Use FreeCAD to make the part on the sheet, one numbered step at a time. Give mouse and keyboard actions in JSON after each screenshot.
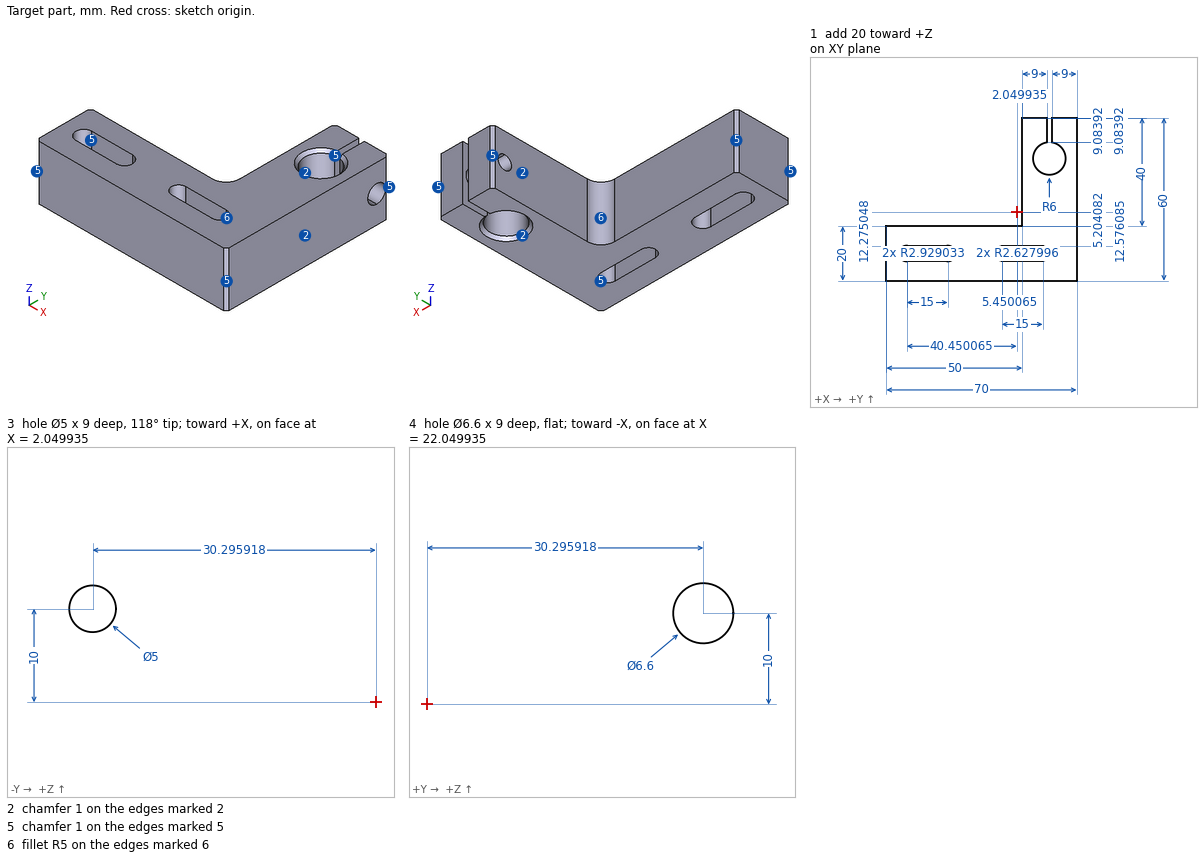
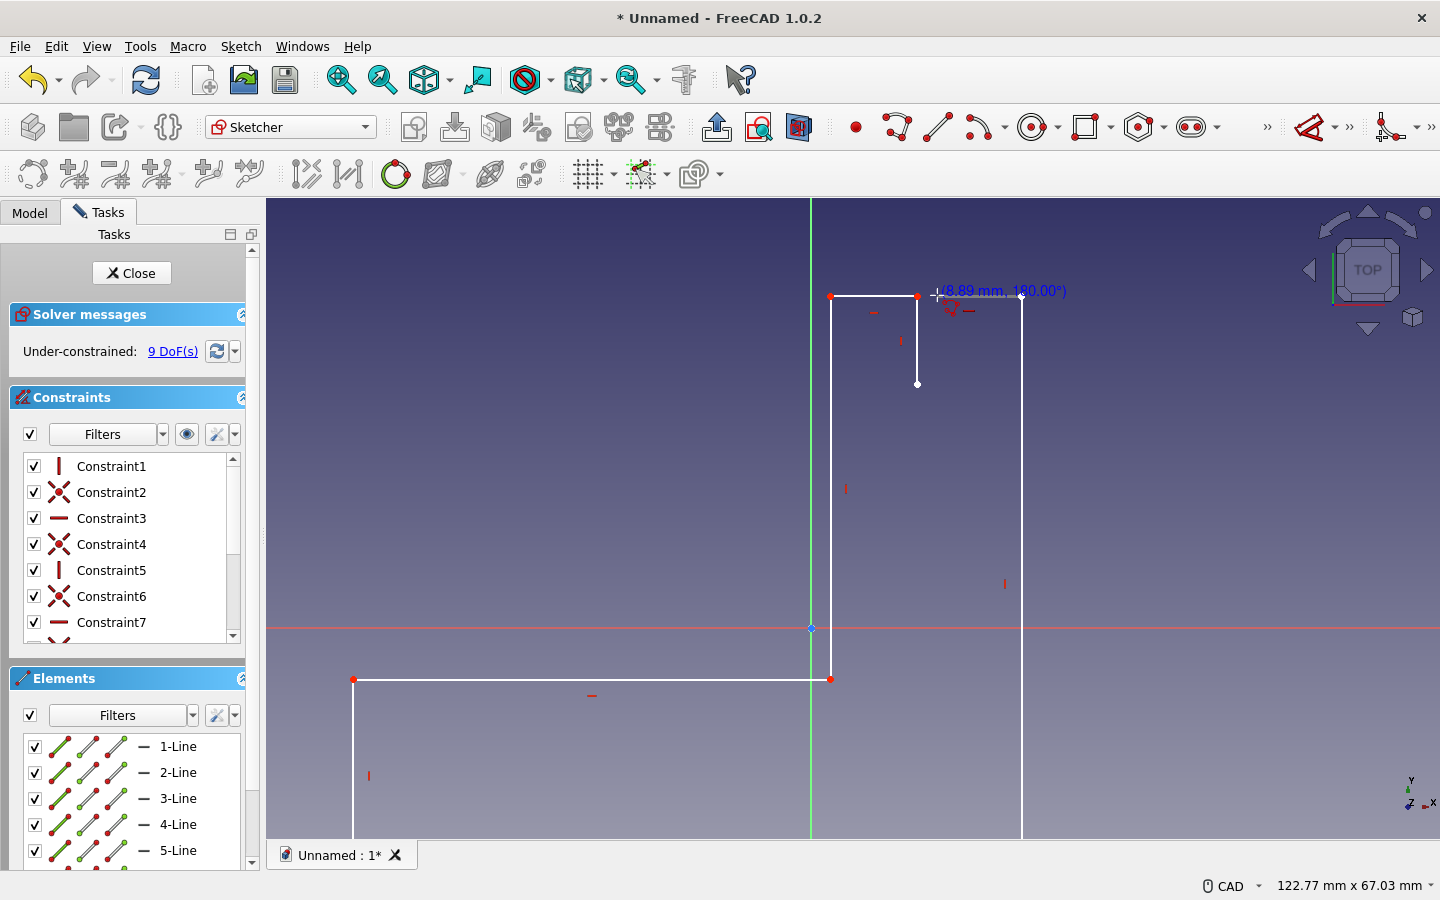
{"action": "left_click", "coordinate": [936, 295]}
{"action": "left_click", "coordinate": [936, 382]}
{"action": "right_click", "coordinate": [936, 382]}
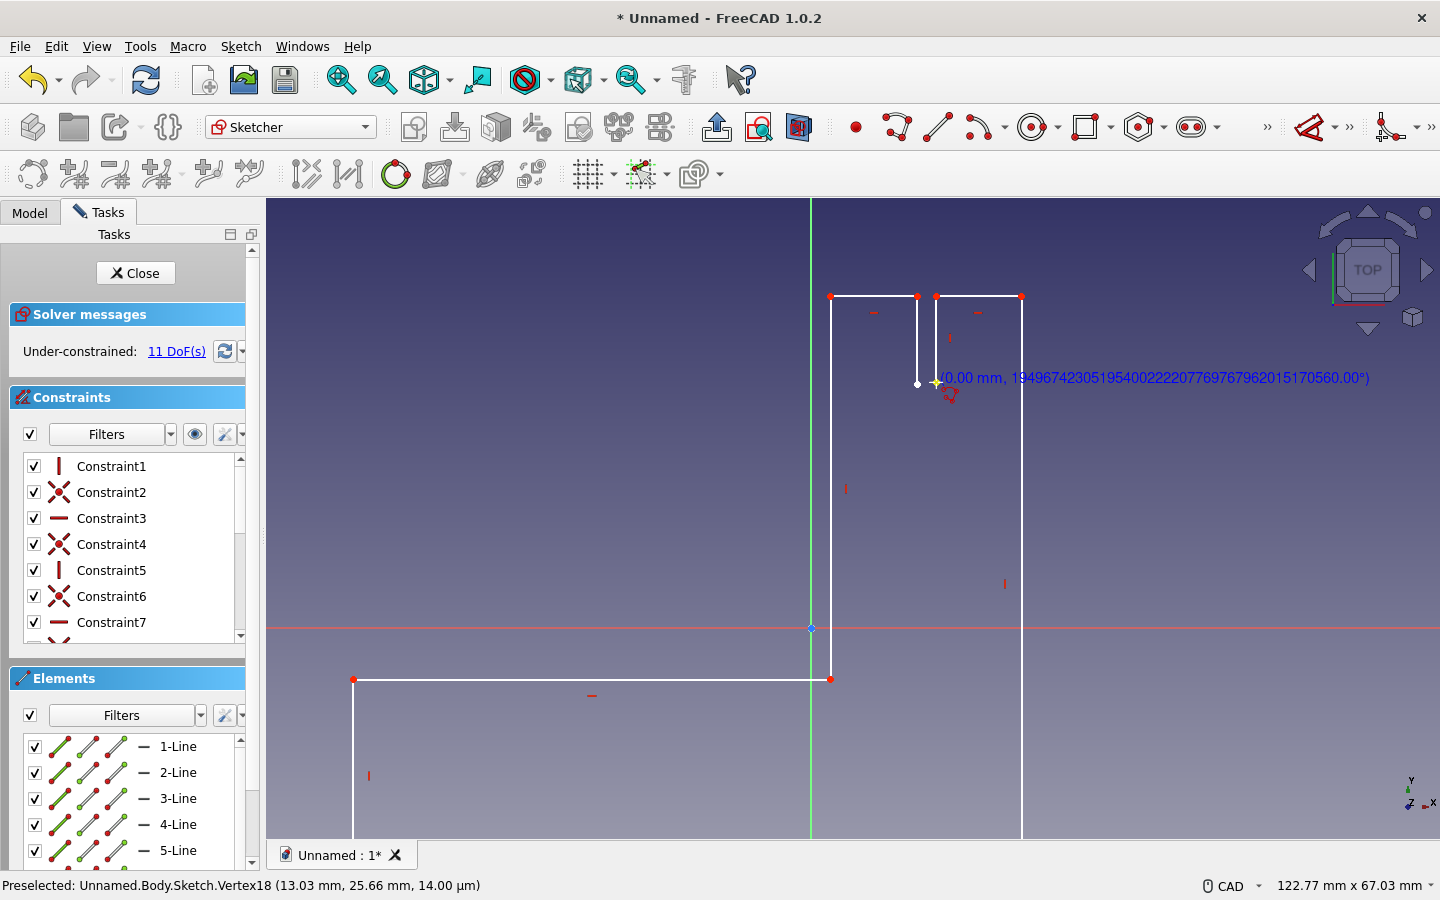
{"action": "left_click", "coordinate": [1004, 128]}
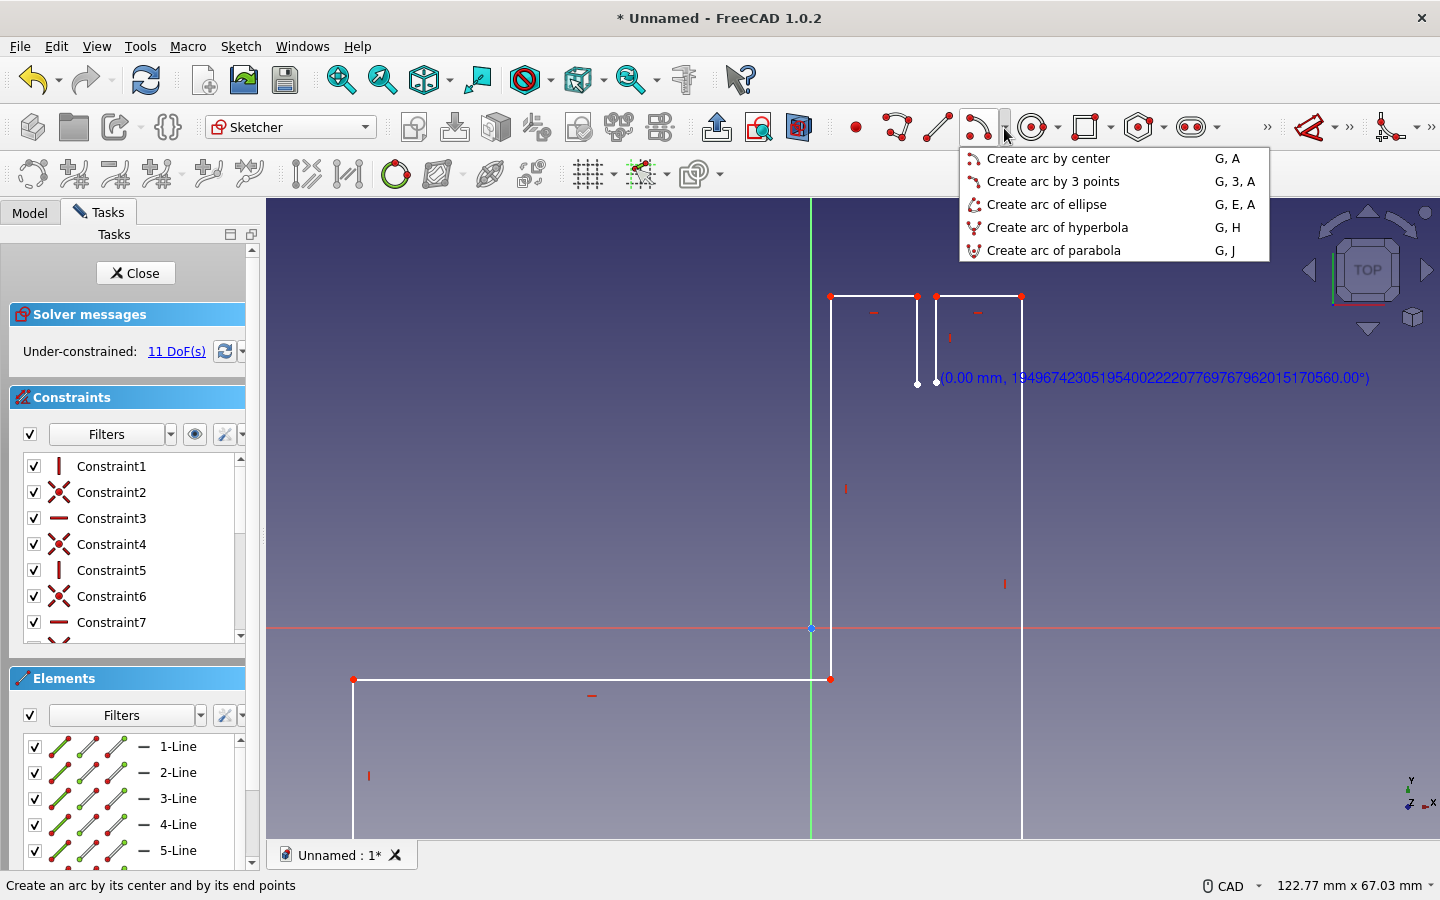
{"action": "left_click", "coordinate": [1114, 182]}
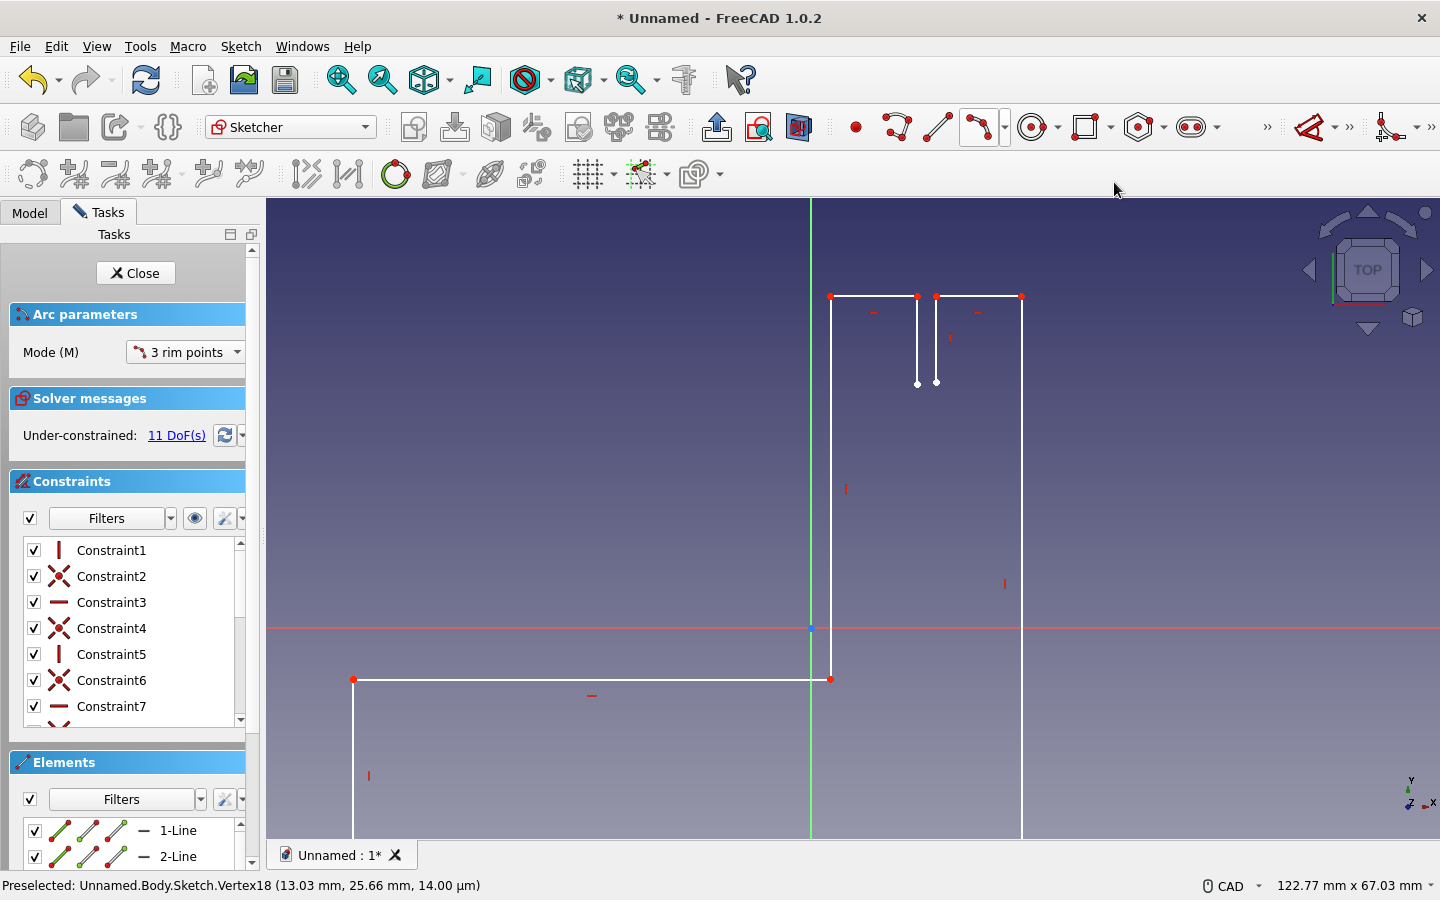
{"action": "left_click", "coordinate": [936, 383]}
{"action": "left_click", "coordinate": [917, 384]}
{"action": "left_click", "coordinate": [927, 496]}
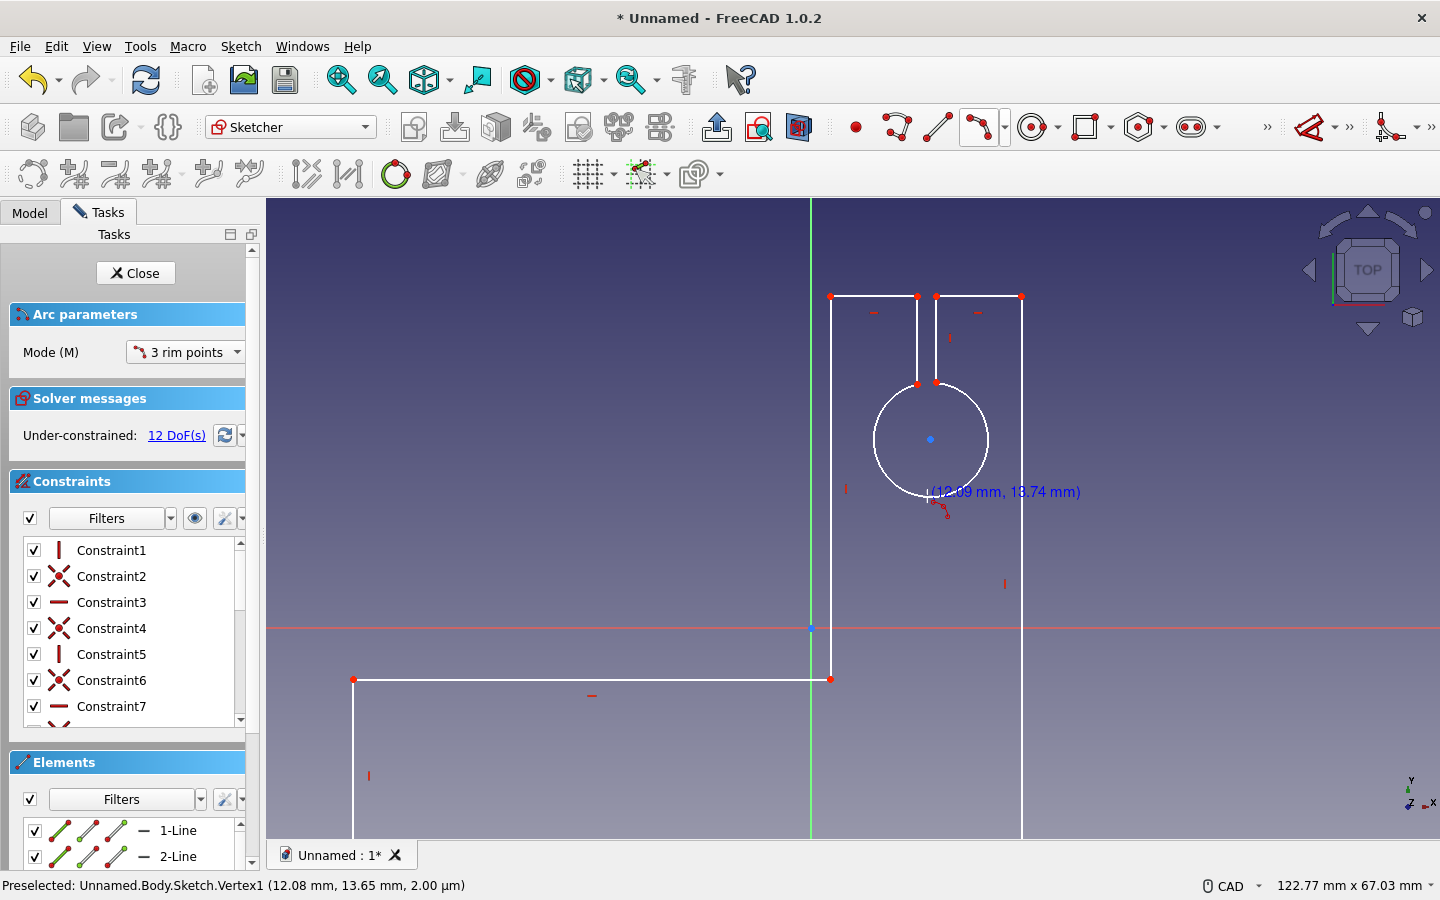
{"action": "left_click", "coordinate": [1190, 128]}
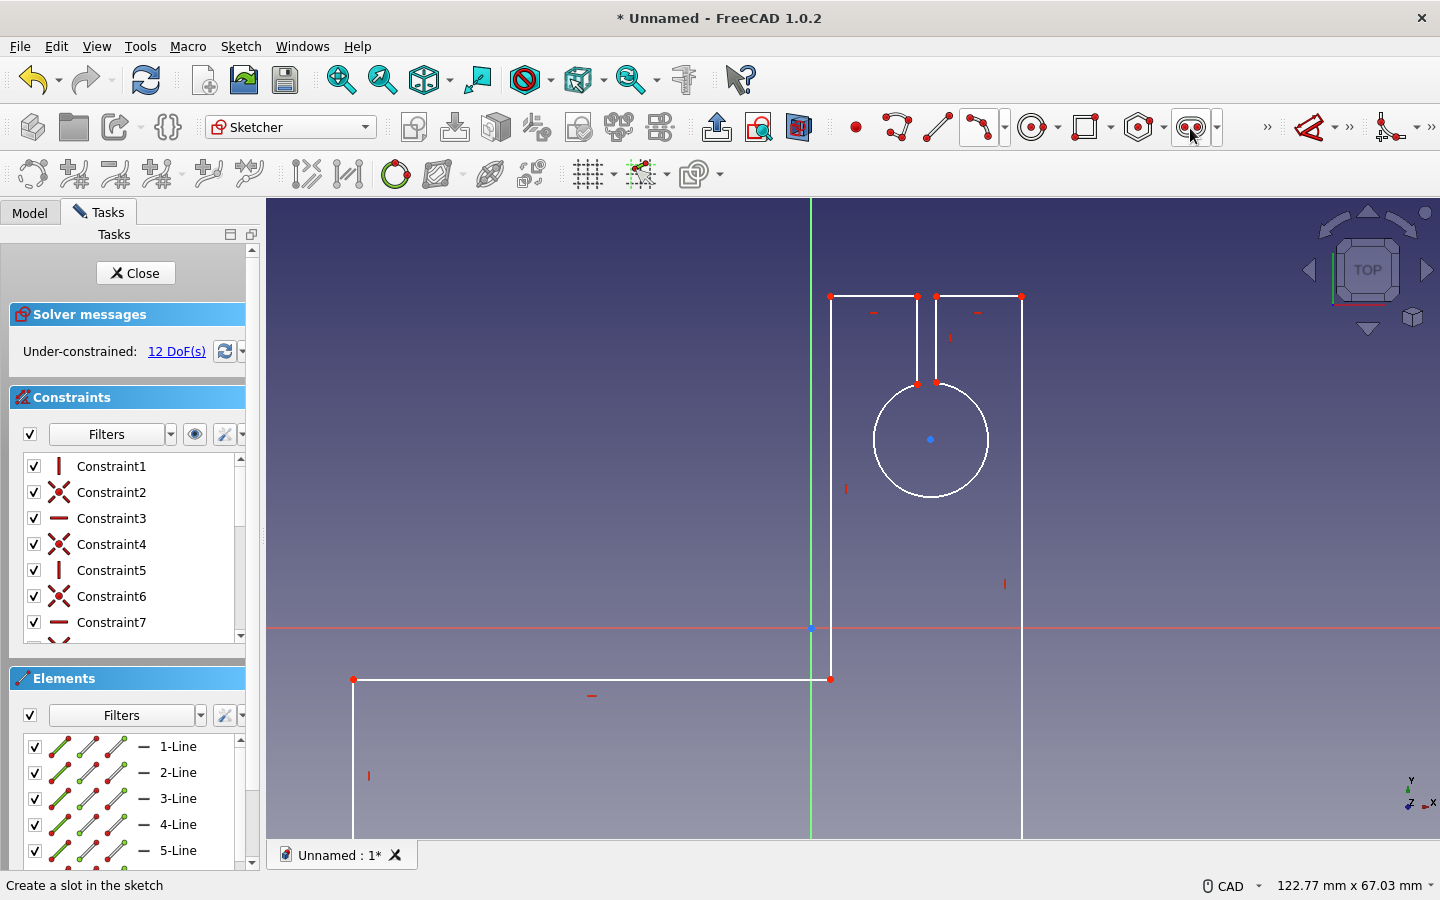
{"action": "left_click", "coordinate": [759, 774]}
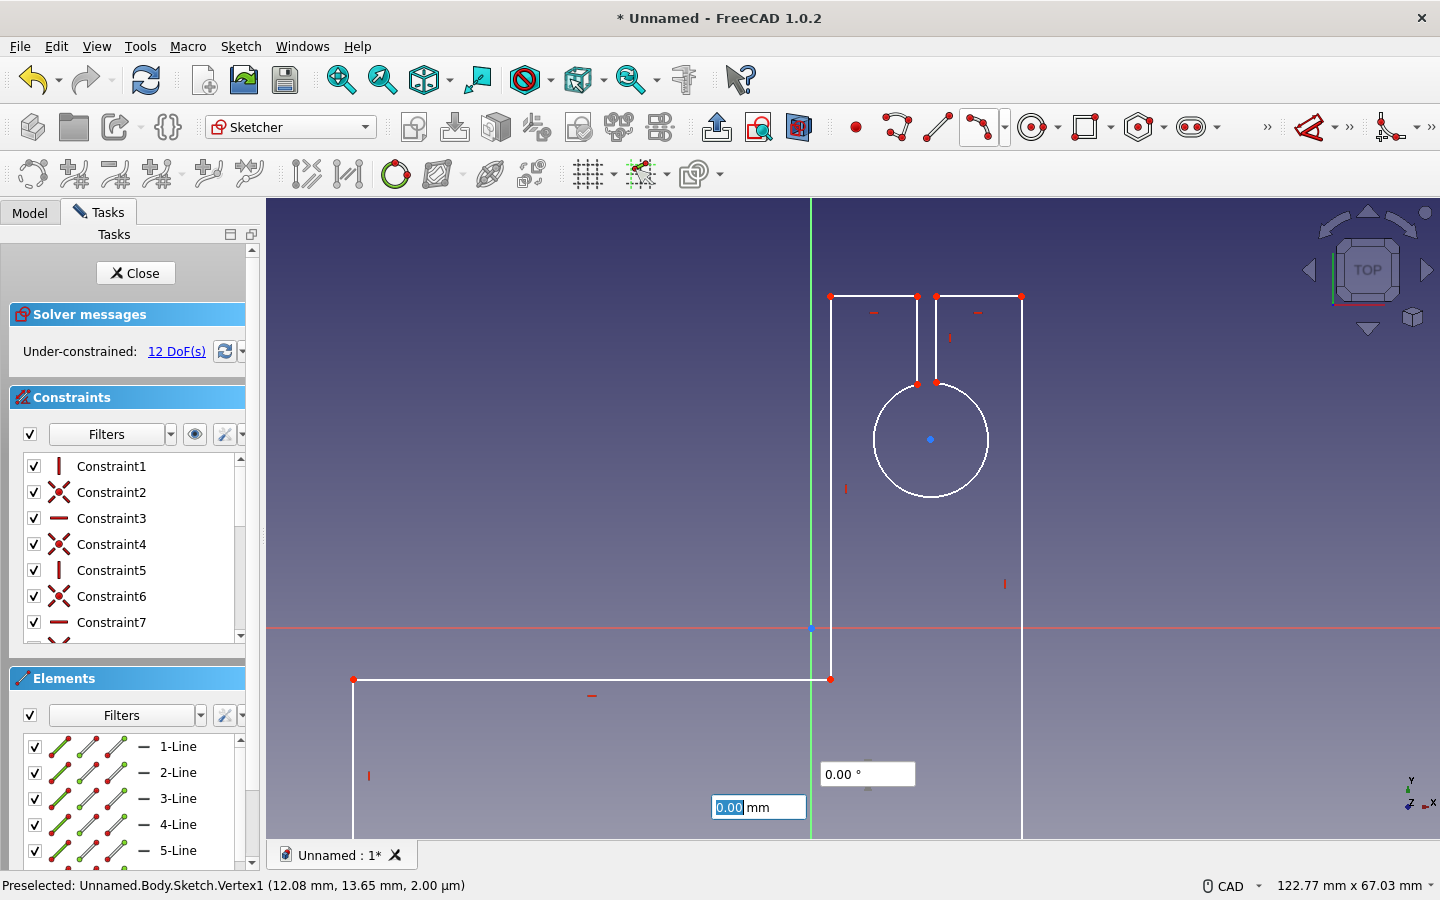
{"action": "left_click", "coordinate": [903, 774]}